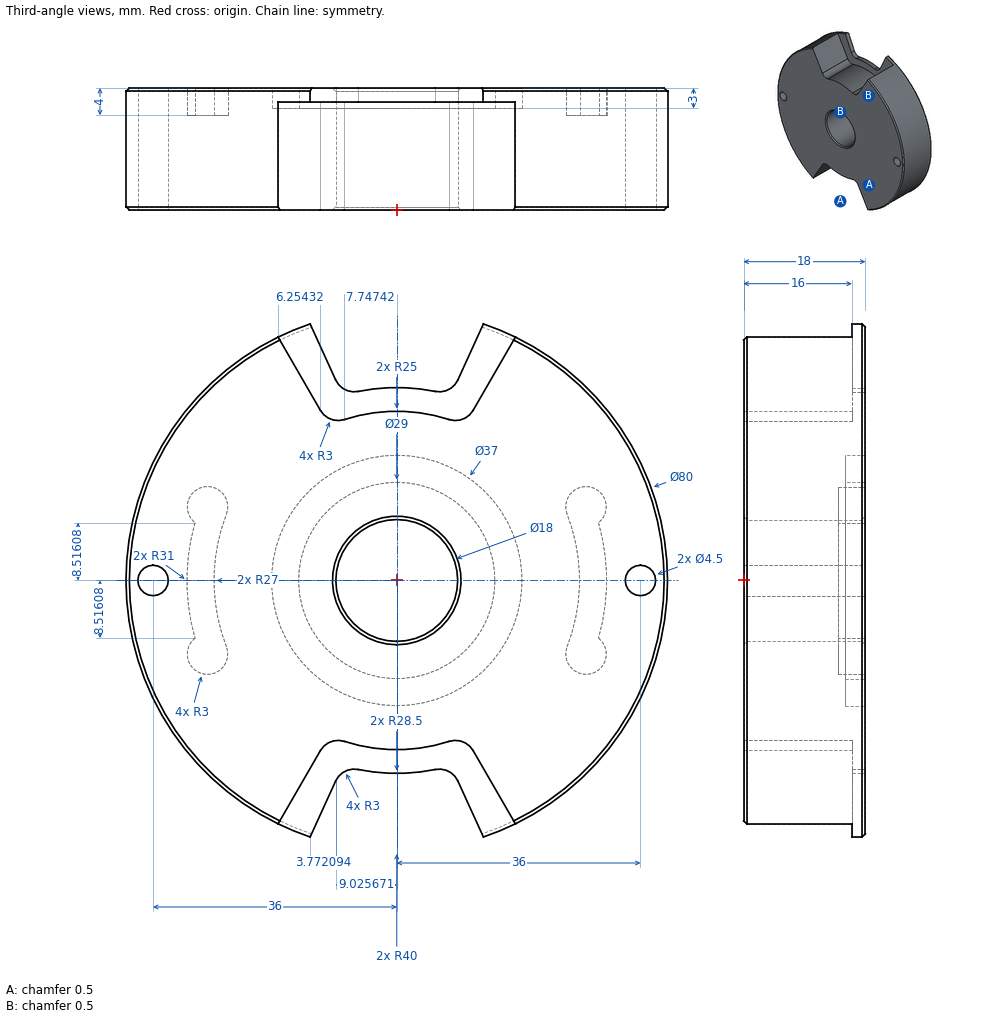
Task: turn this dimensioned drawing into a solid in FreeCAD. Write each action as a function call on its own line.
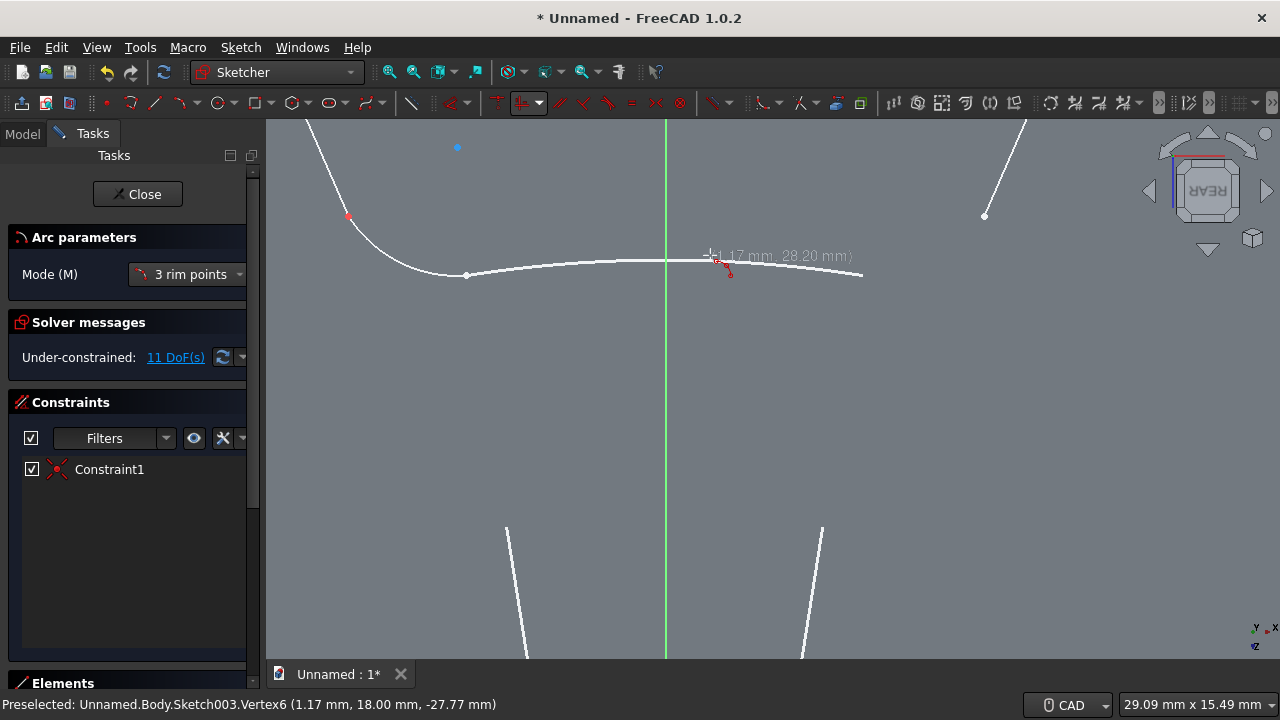
click(706, 251)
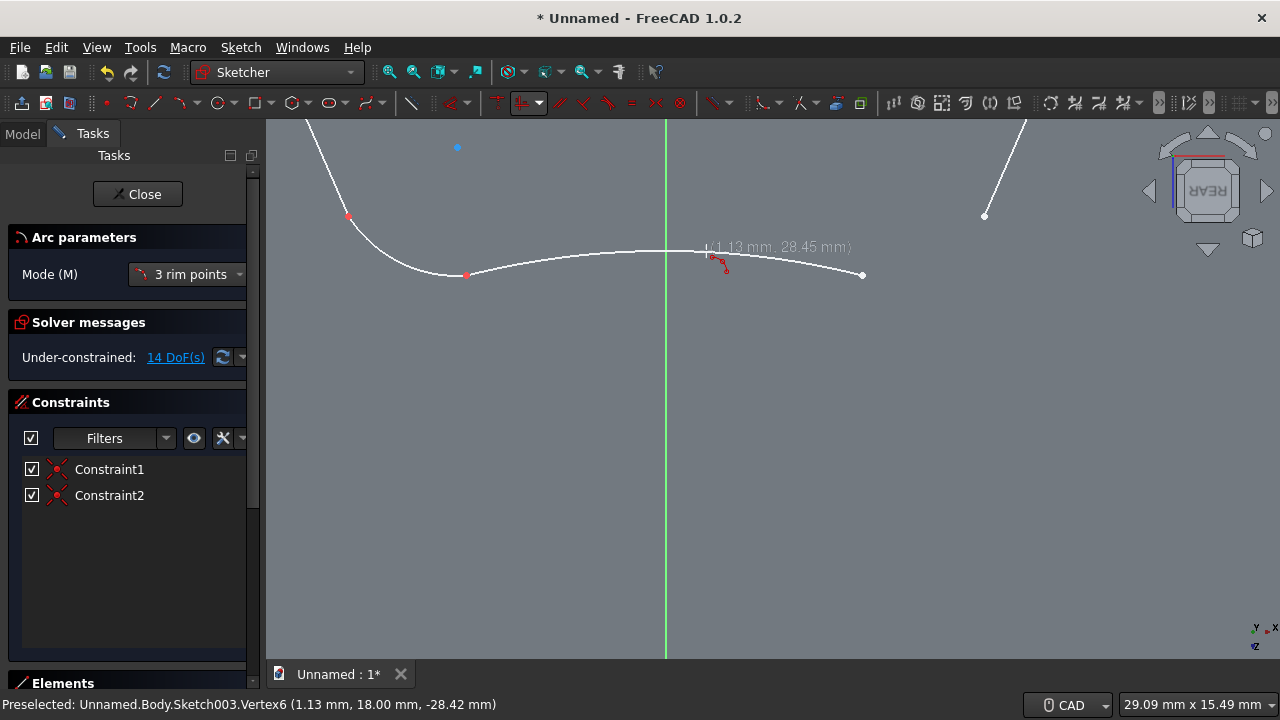
scroll(710, 255, down, 10)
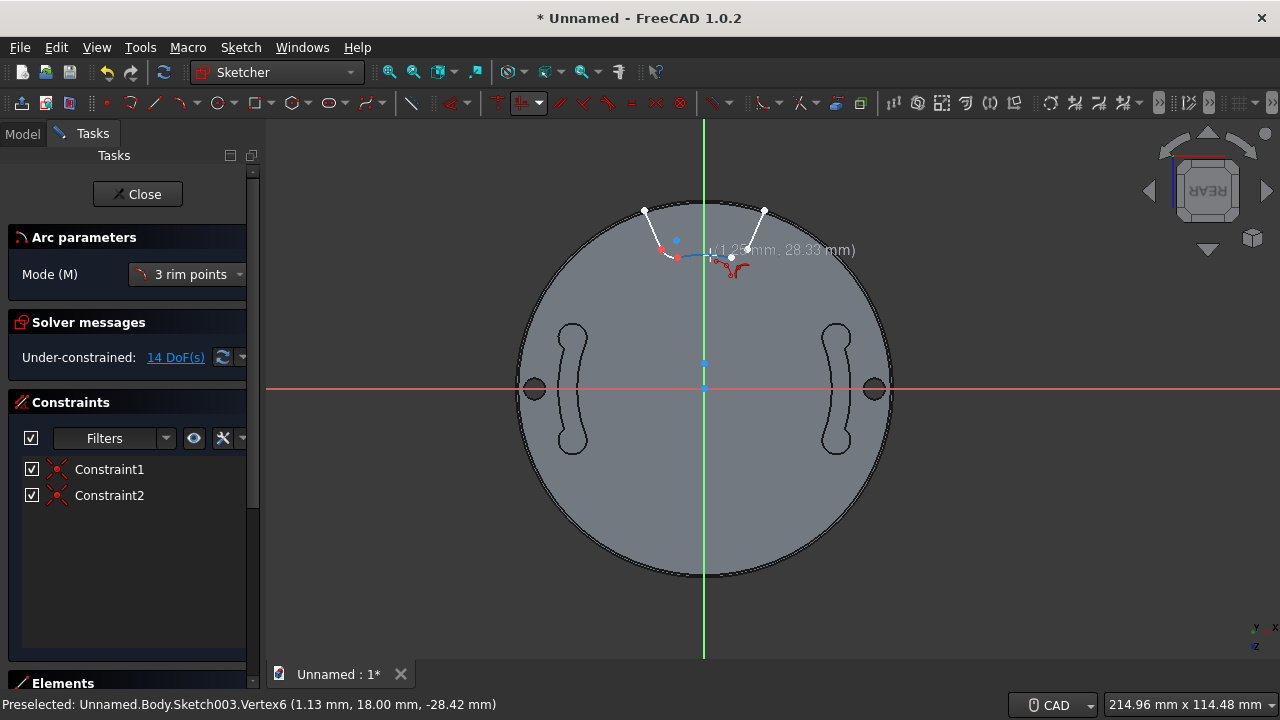
click(731, 258)
click(747, 250)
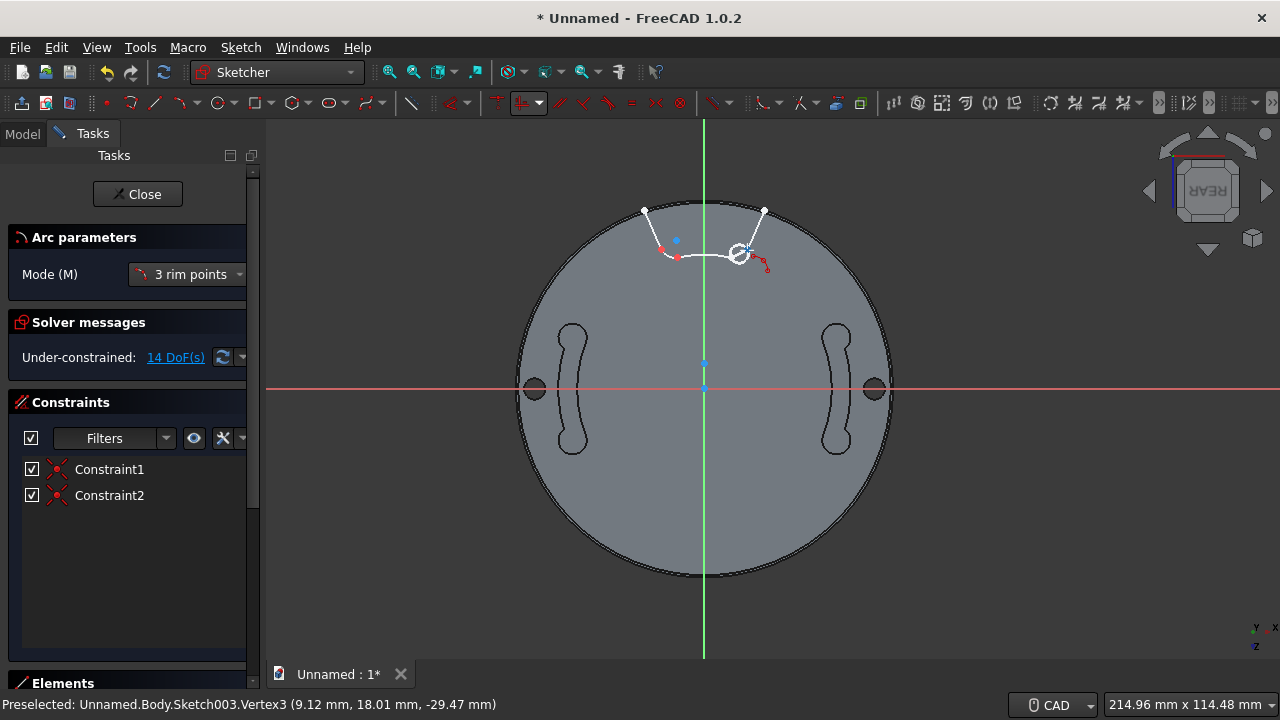
scroll(741, 256, up, 9)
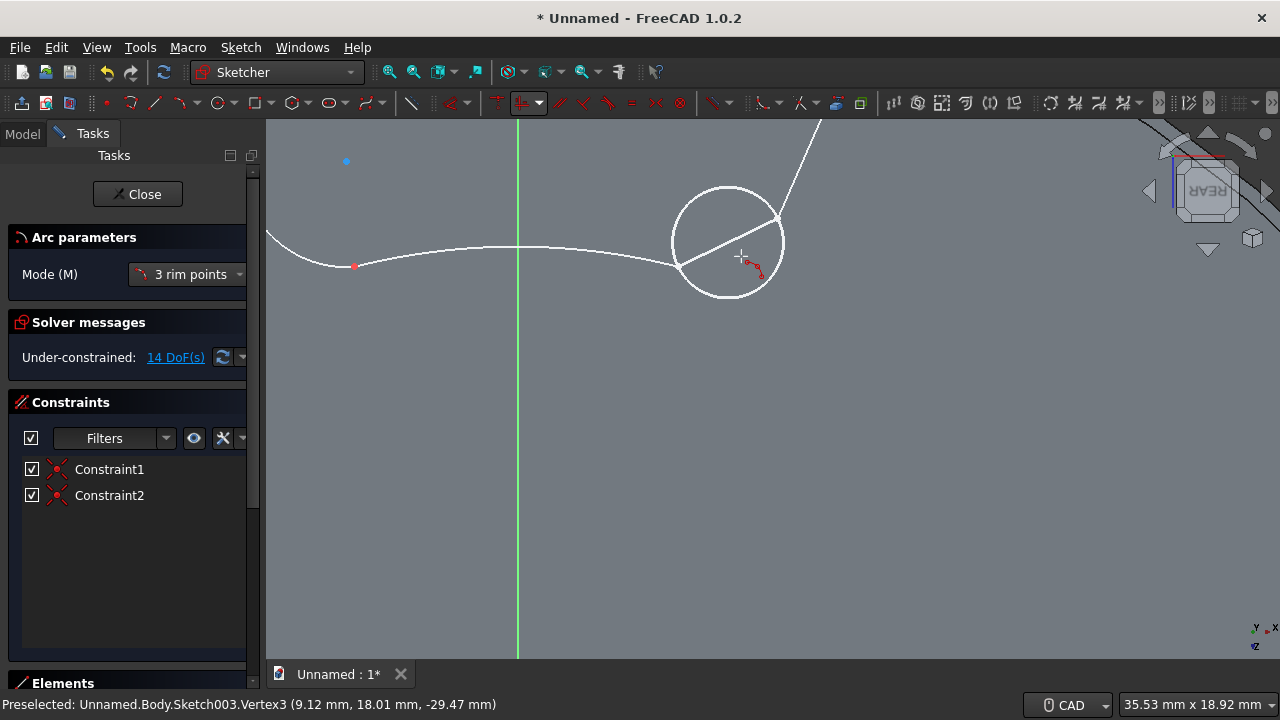
click(736, 255)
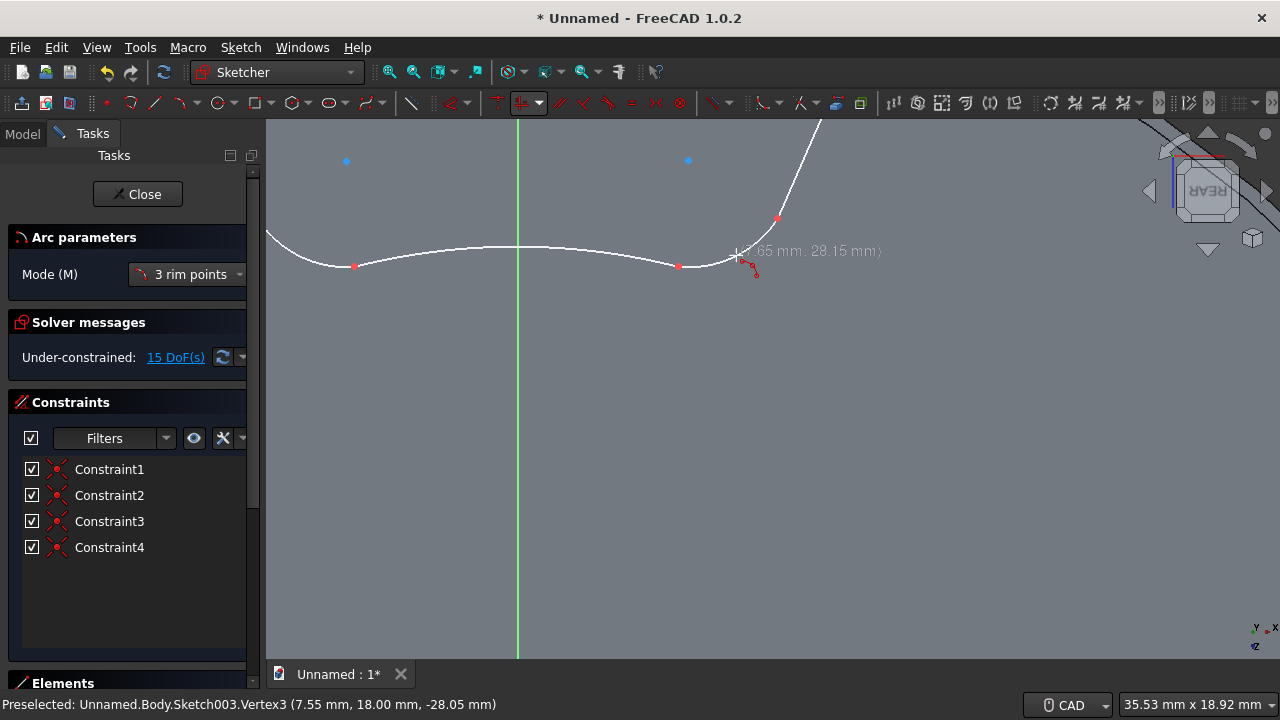
scroll(741, 256, down, 9)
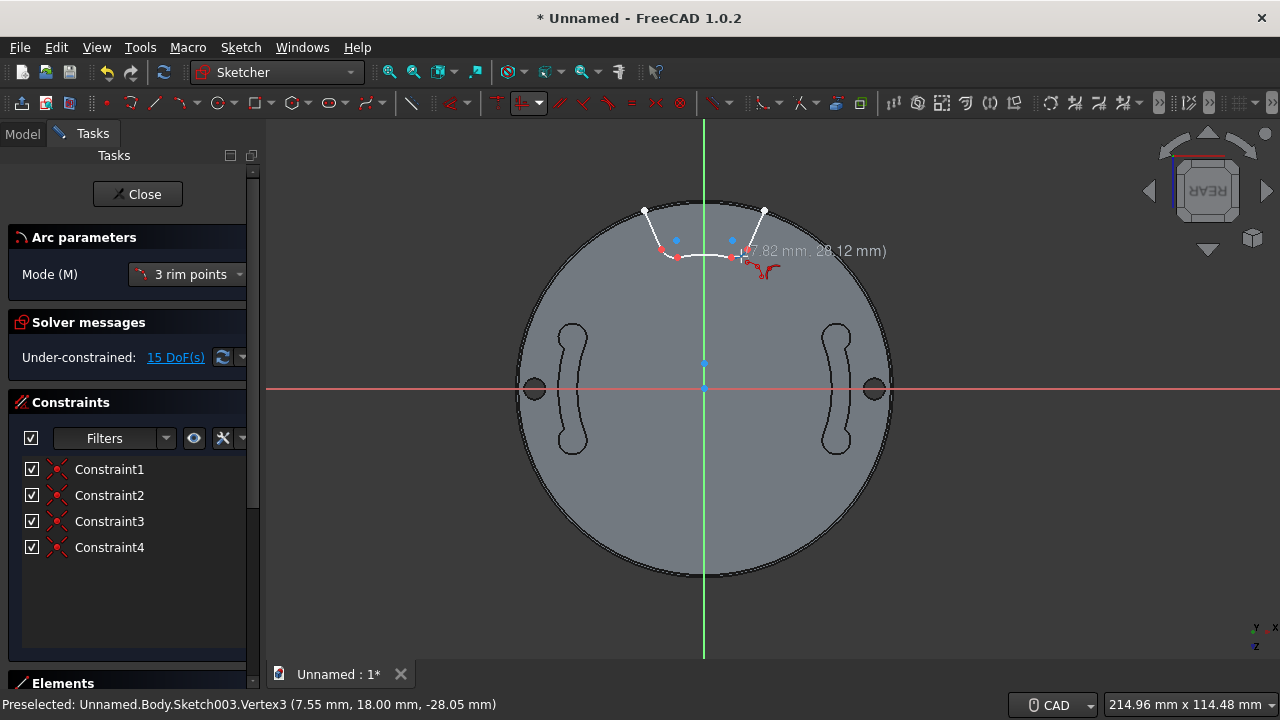
click(764, 211)
click(644, 211)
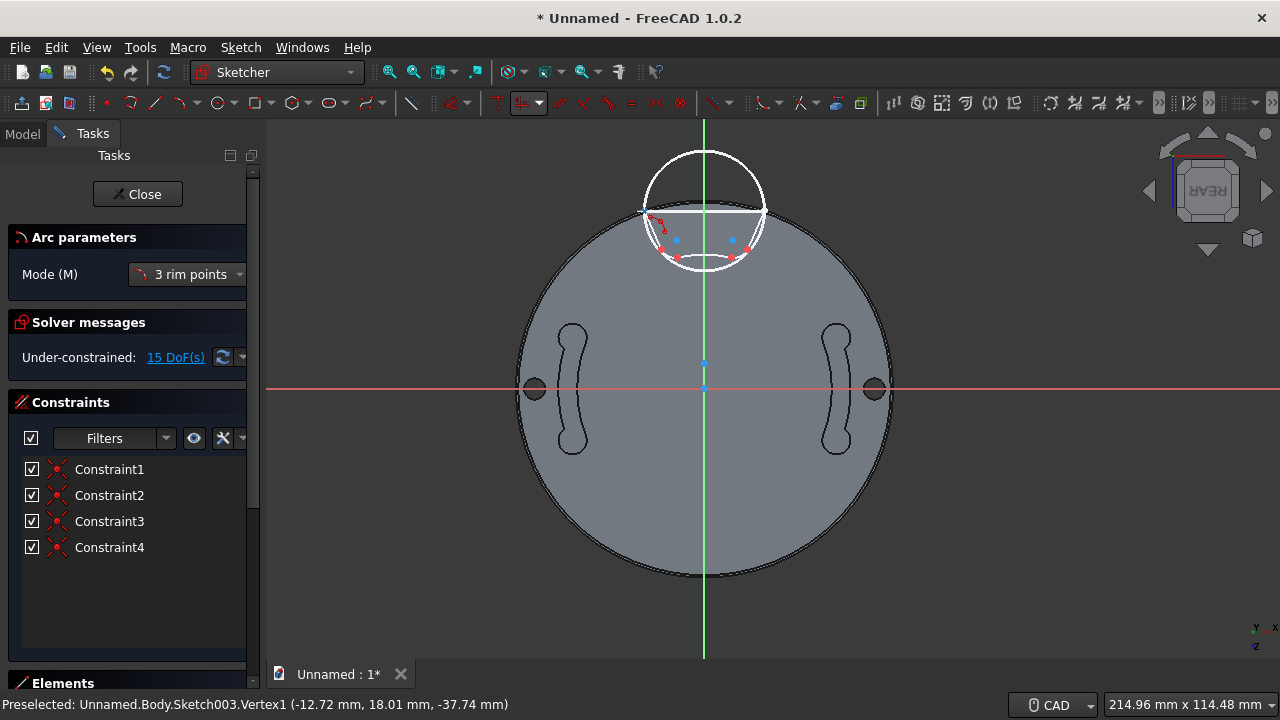
scroll(717, 201, up, 3)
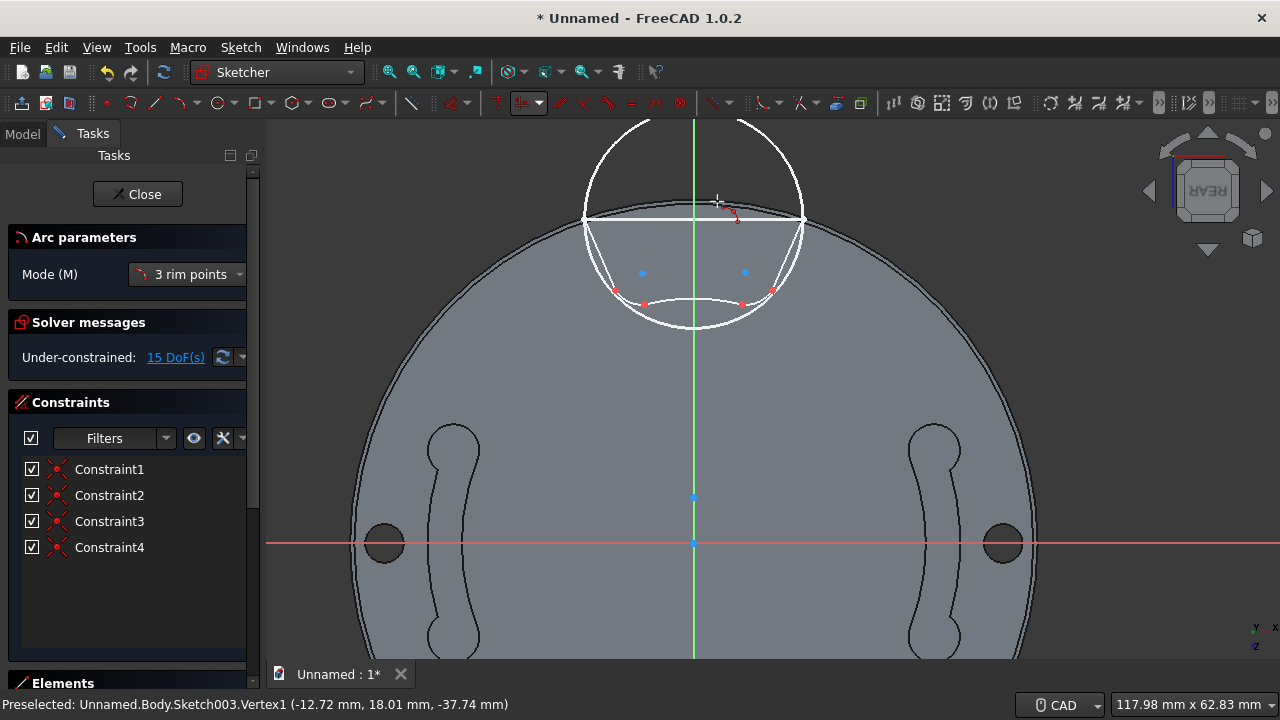
click(716, 200)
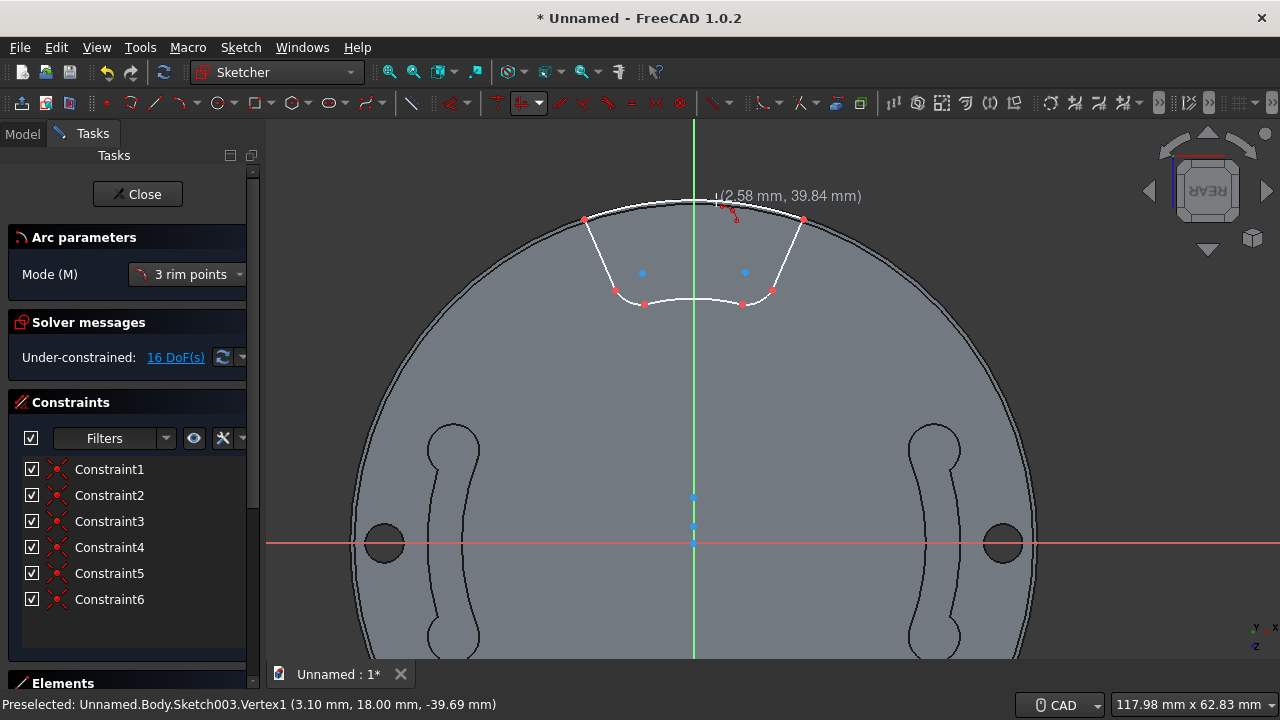
click(156, 104)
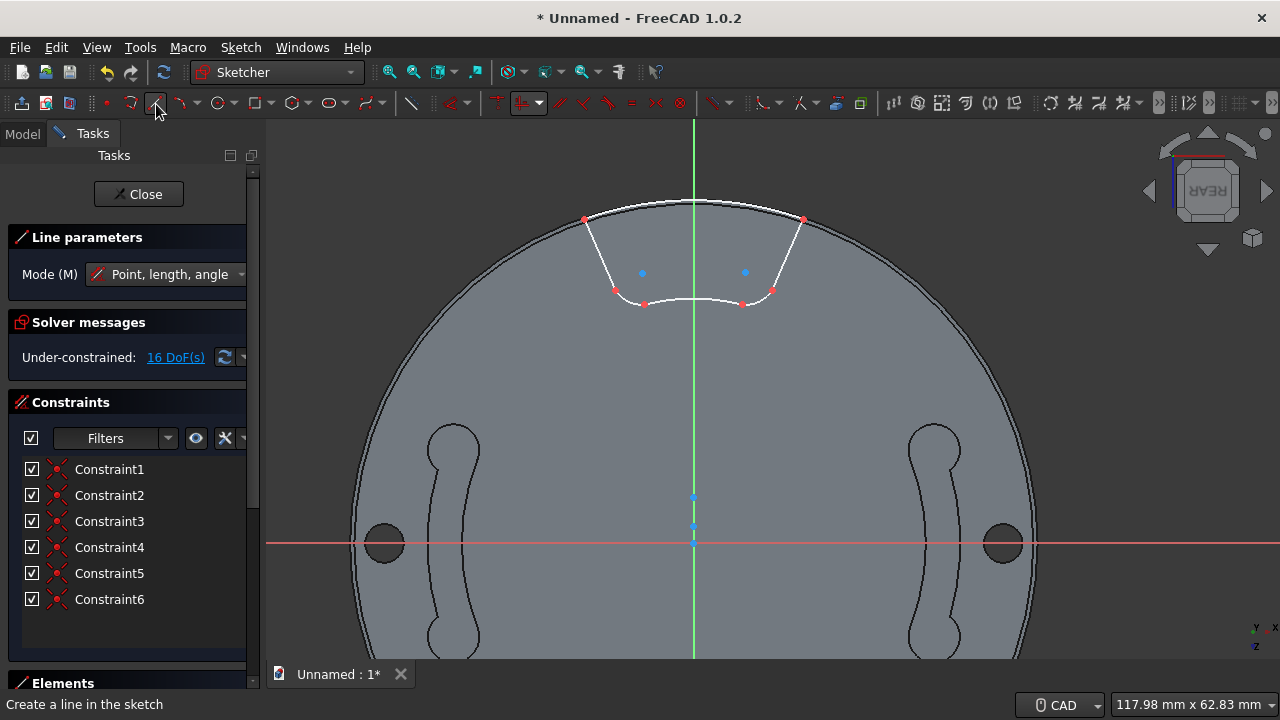
scroll(717, 201, down, 3)